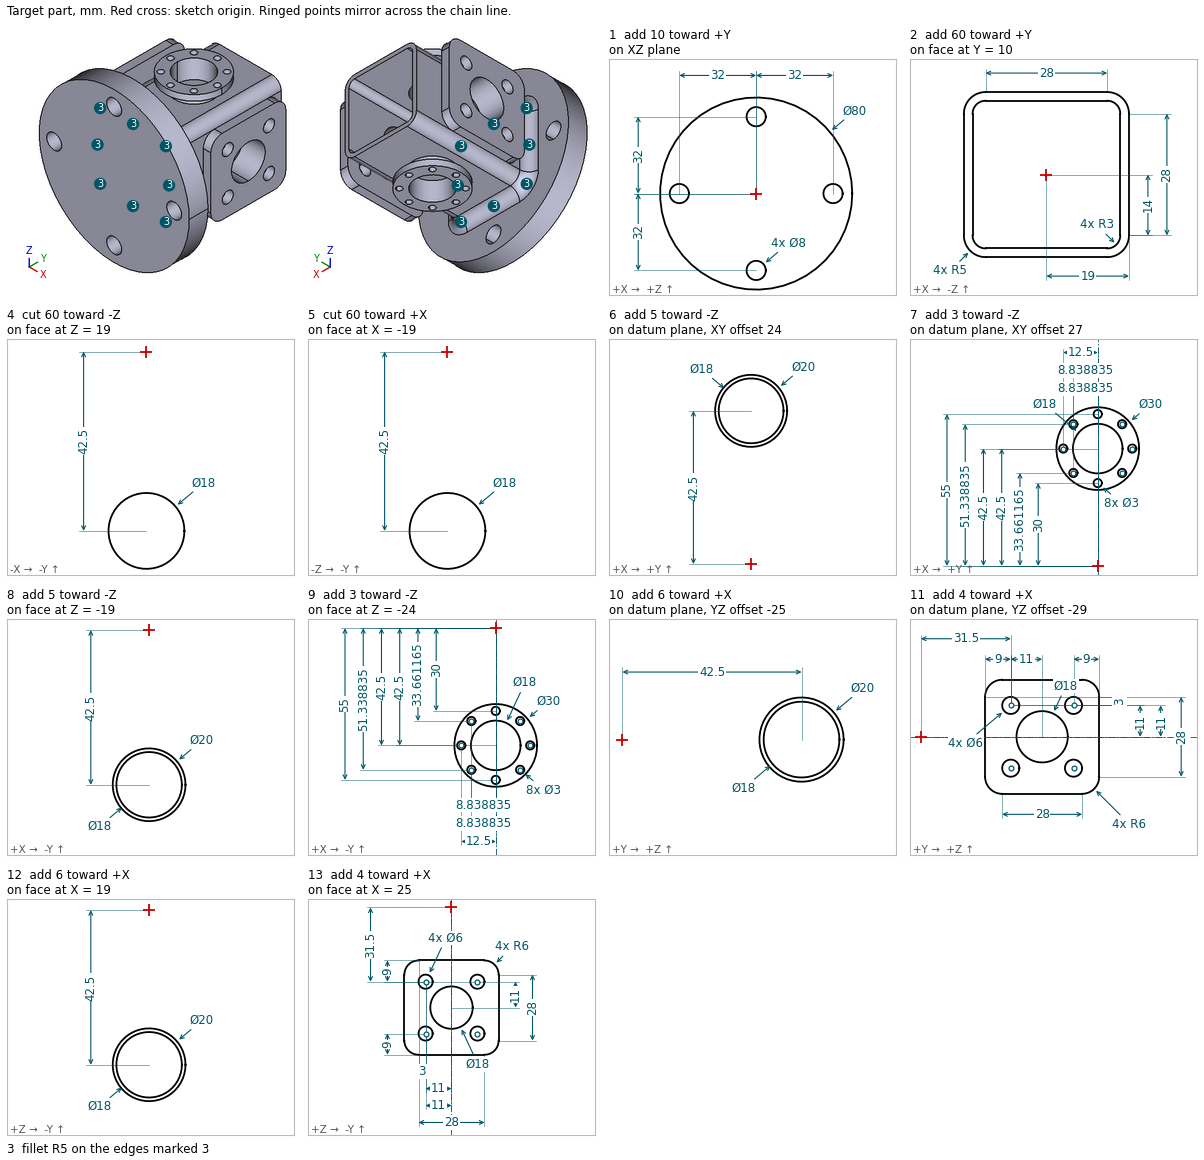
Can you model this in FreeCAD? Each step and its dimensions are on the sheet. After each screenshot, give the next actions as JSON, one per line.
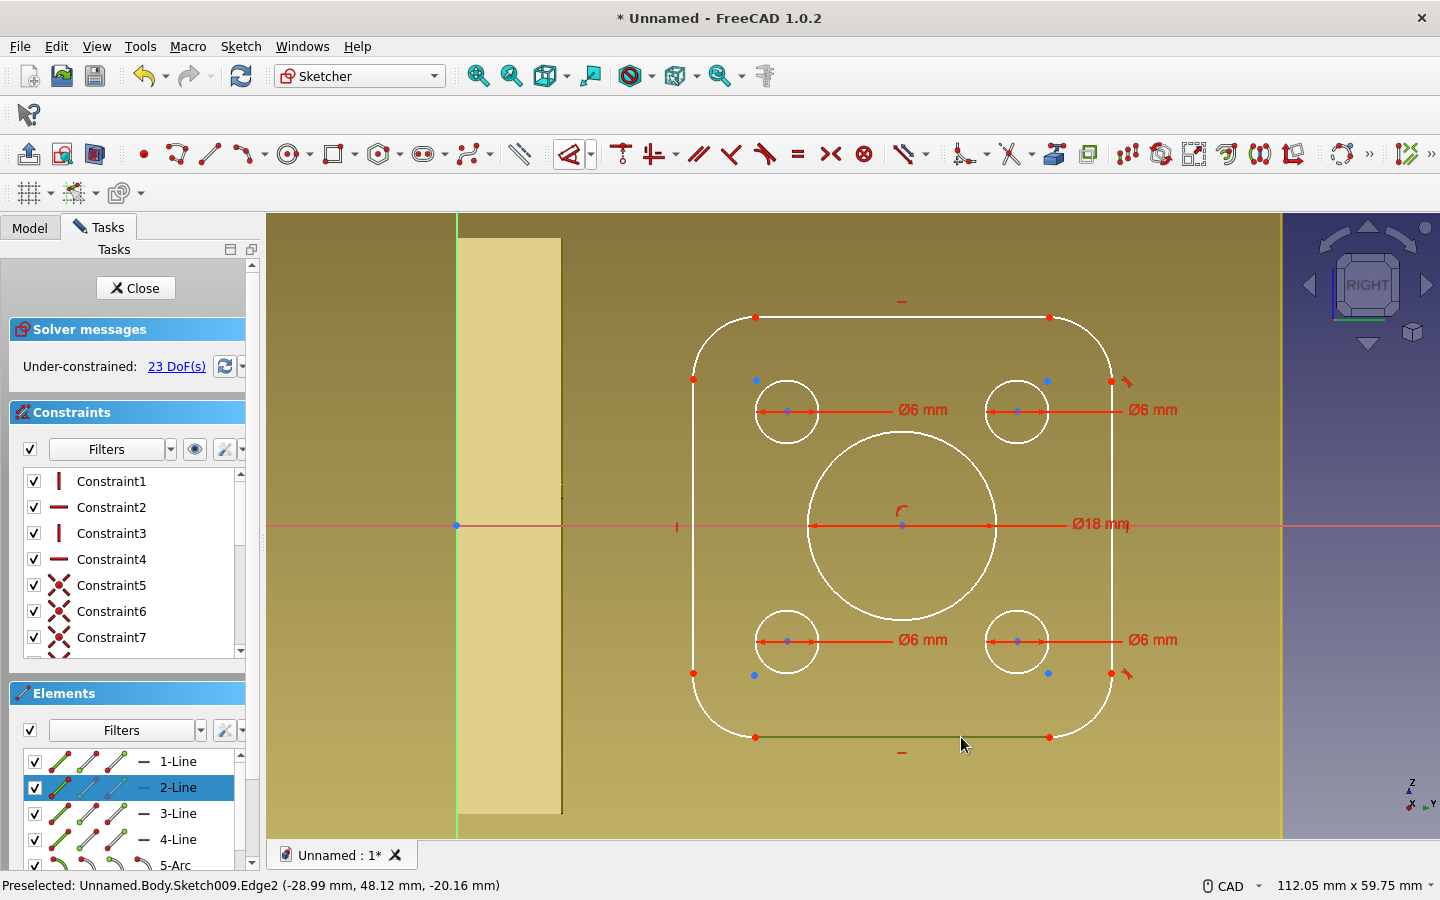
{"action": "left_click", "coordinate": [1078, 730]}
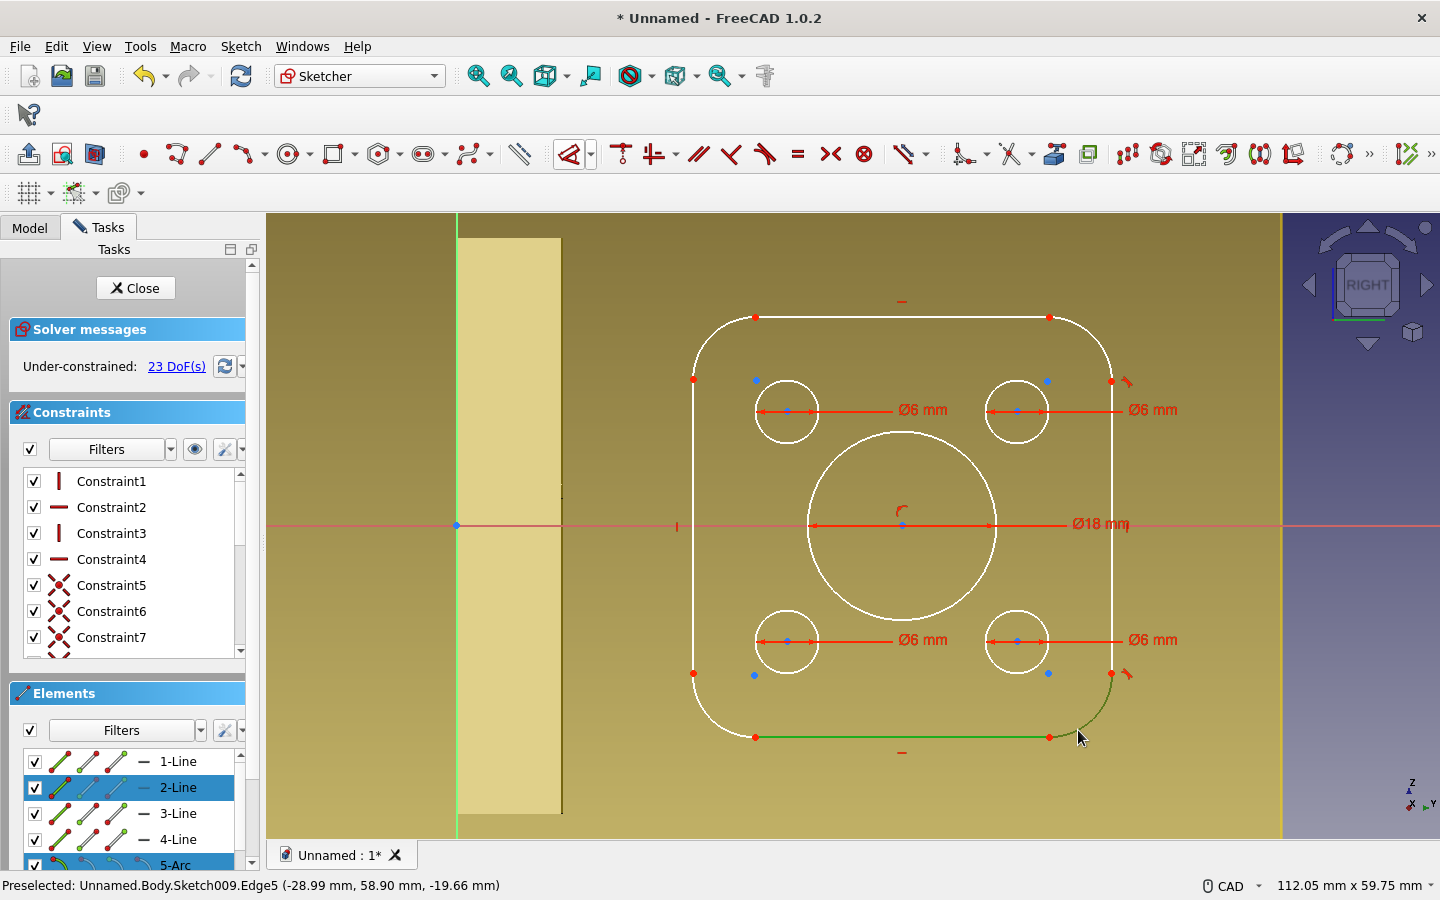
{"action": "left_click", "coordinate": [765, 154]}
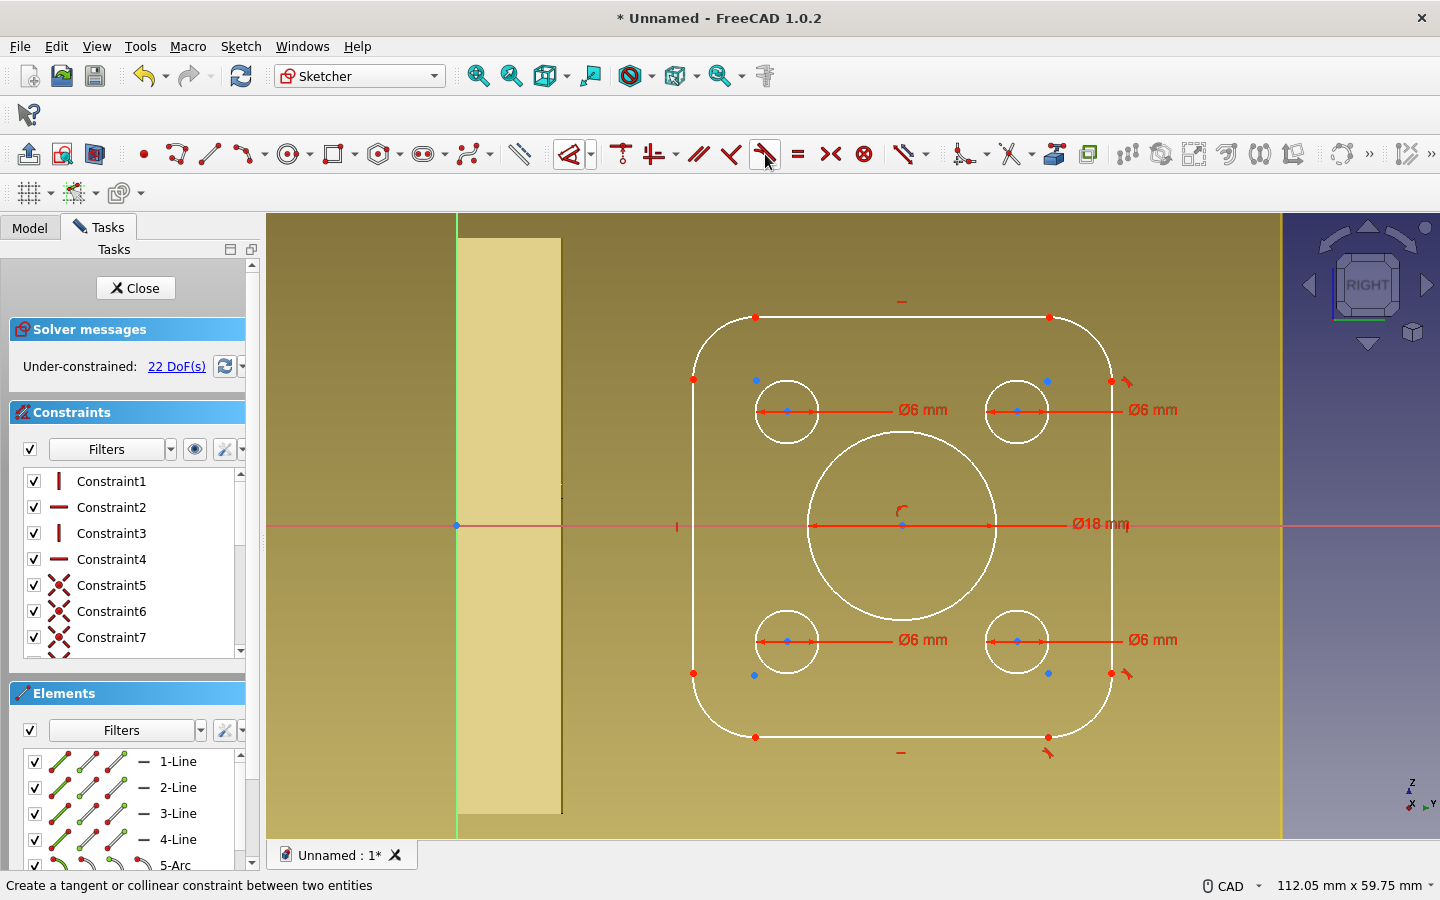
{"action": "left_click", "coordinate": [961, 737]}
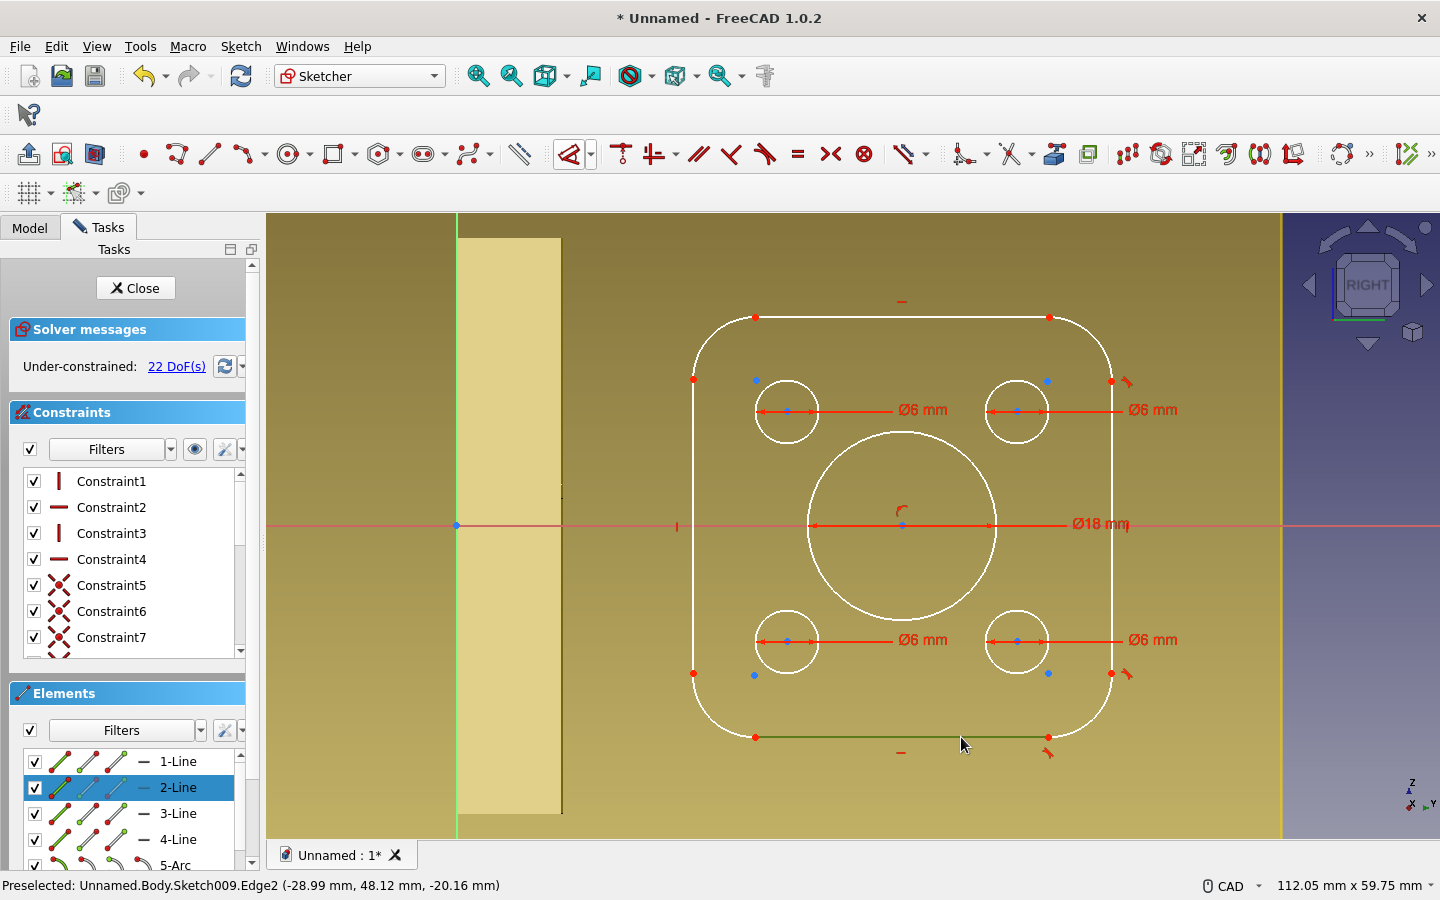
{"action": "left_click", "coordinate": [699, 703]}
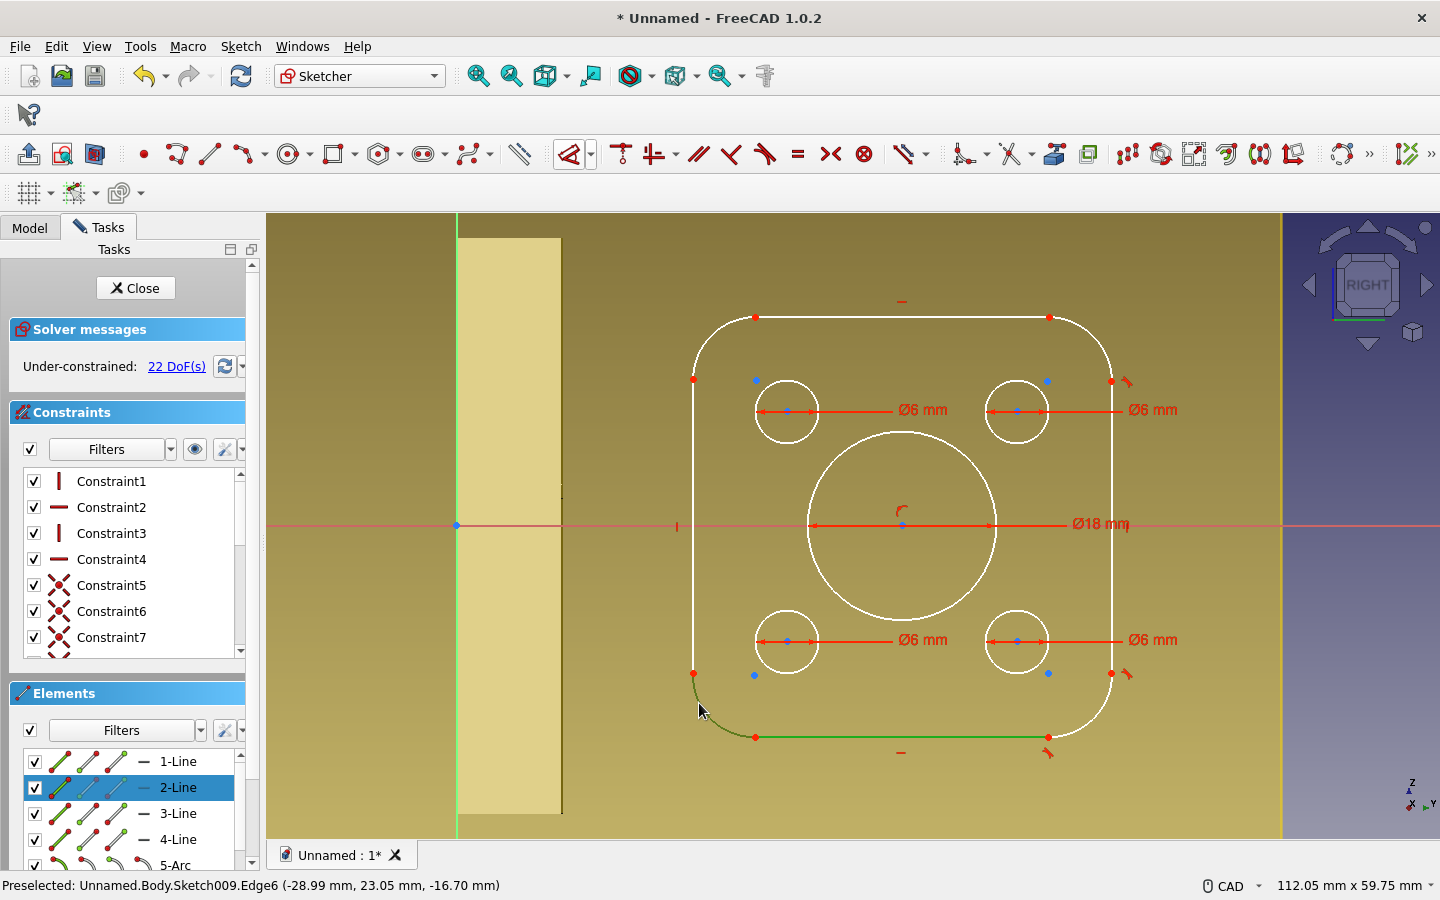
{"action": "key", "text": "t"}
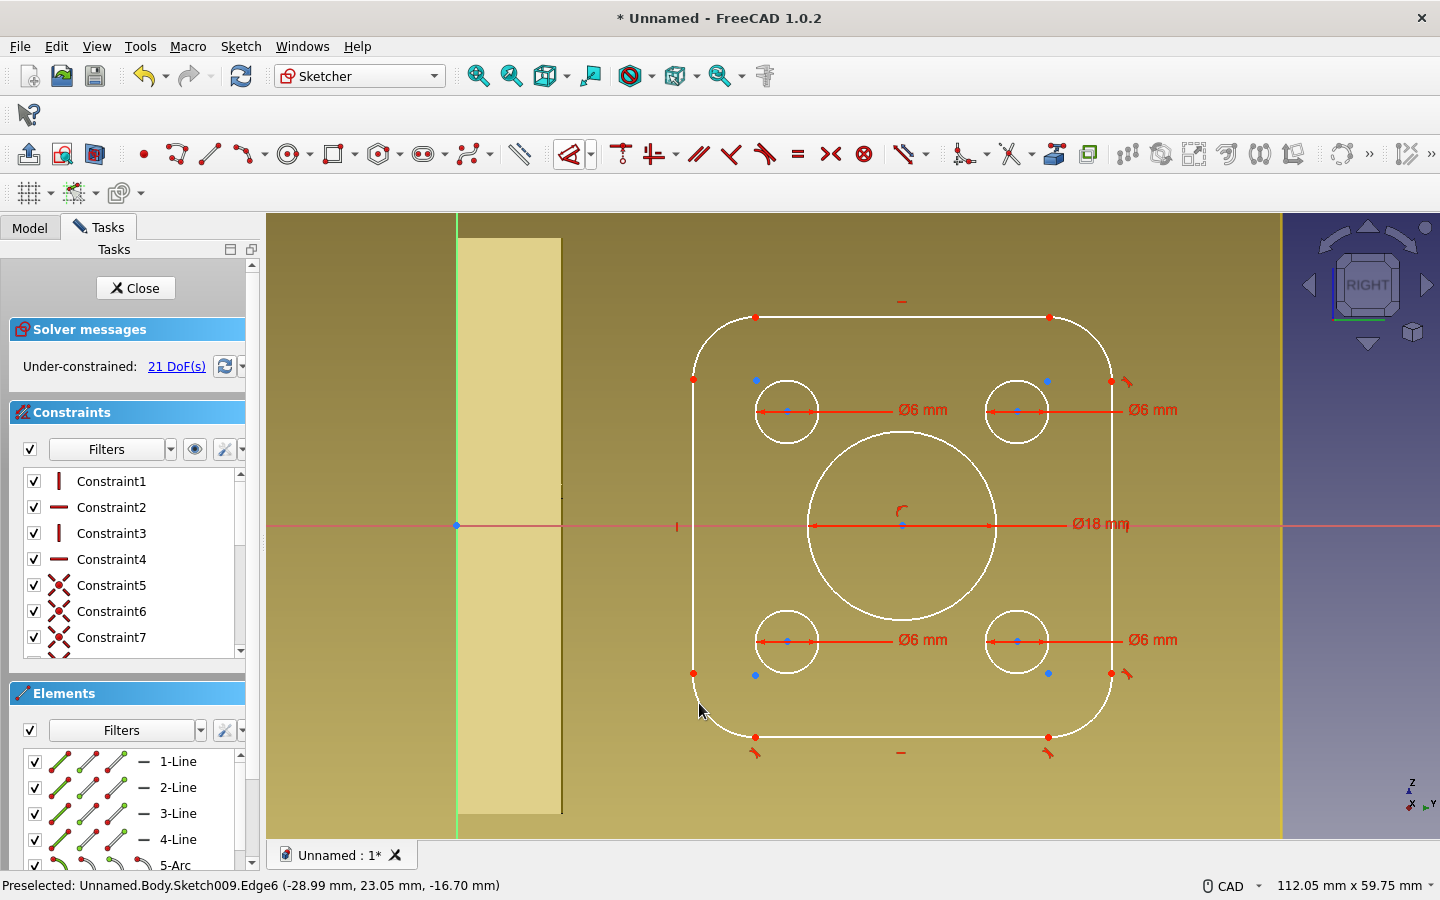
{"action": "left_click", "coordinate": [693, 586]}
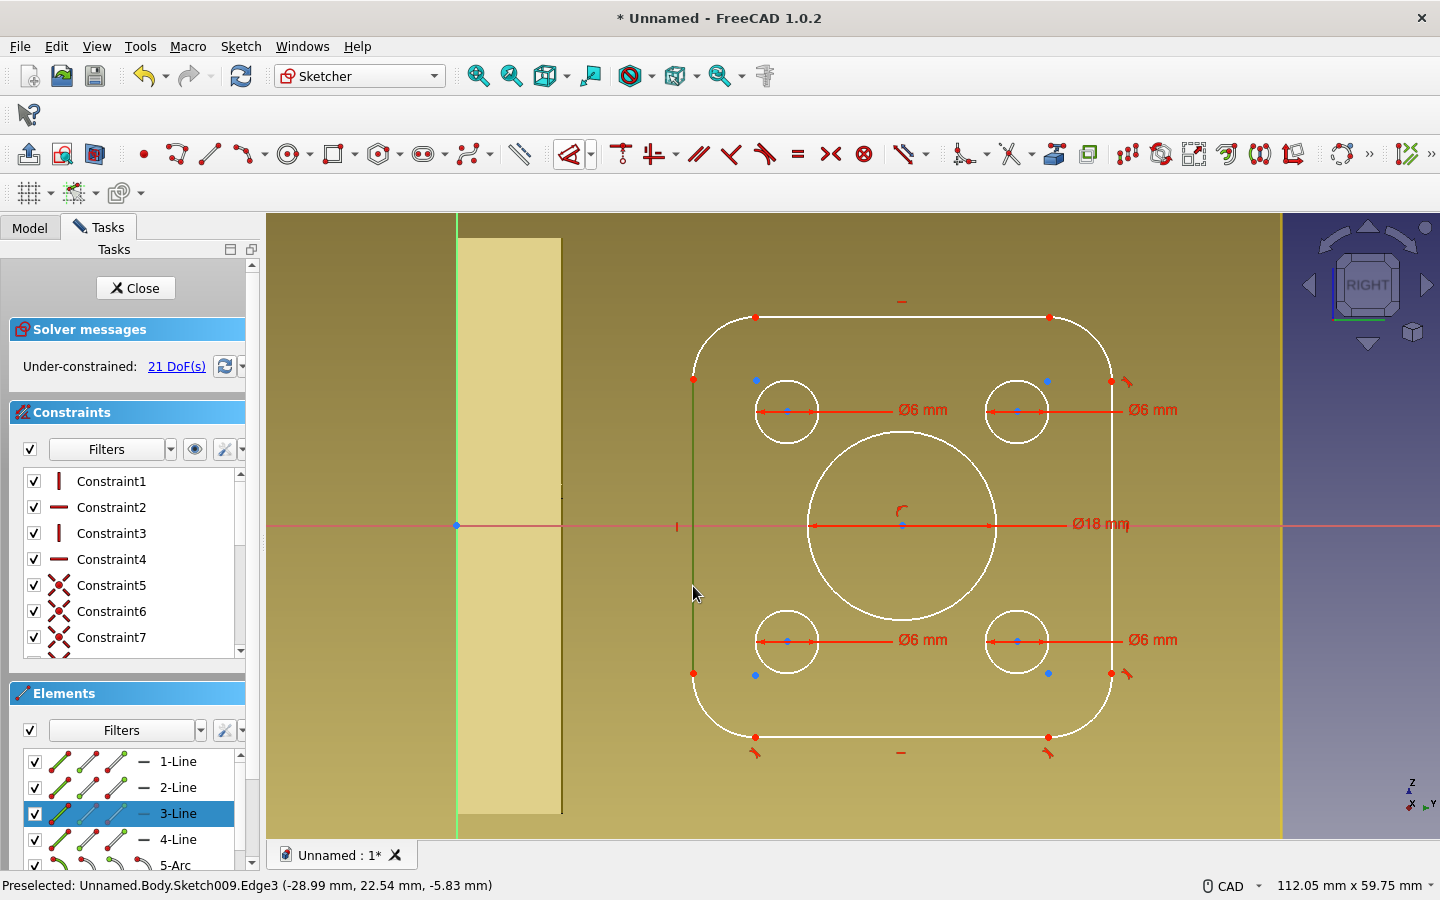
{"action": "left_click", "coordinate": [699, 703]}